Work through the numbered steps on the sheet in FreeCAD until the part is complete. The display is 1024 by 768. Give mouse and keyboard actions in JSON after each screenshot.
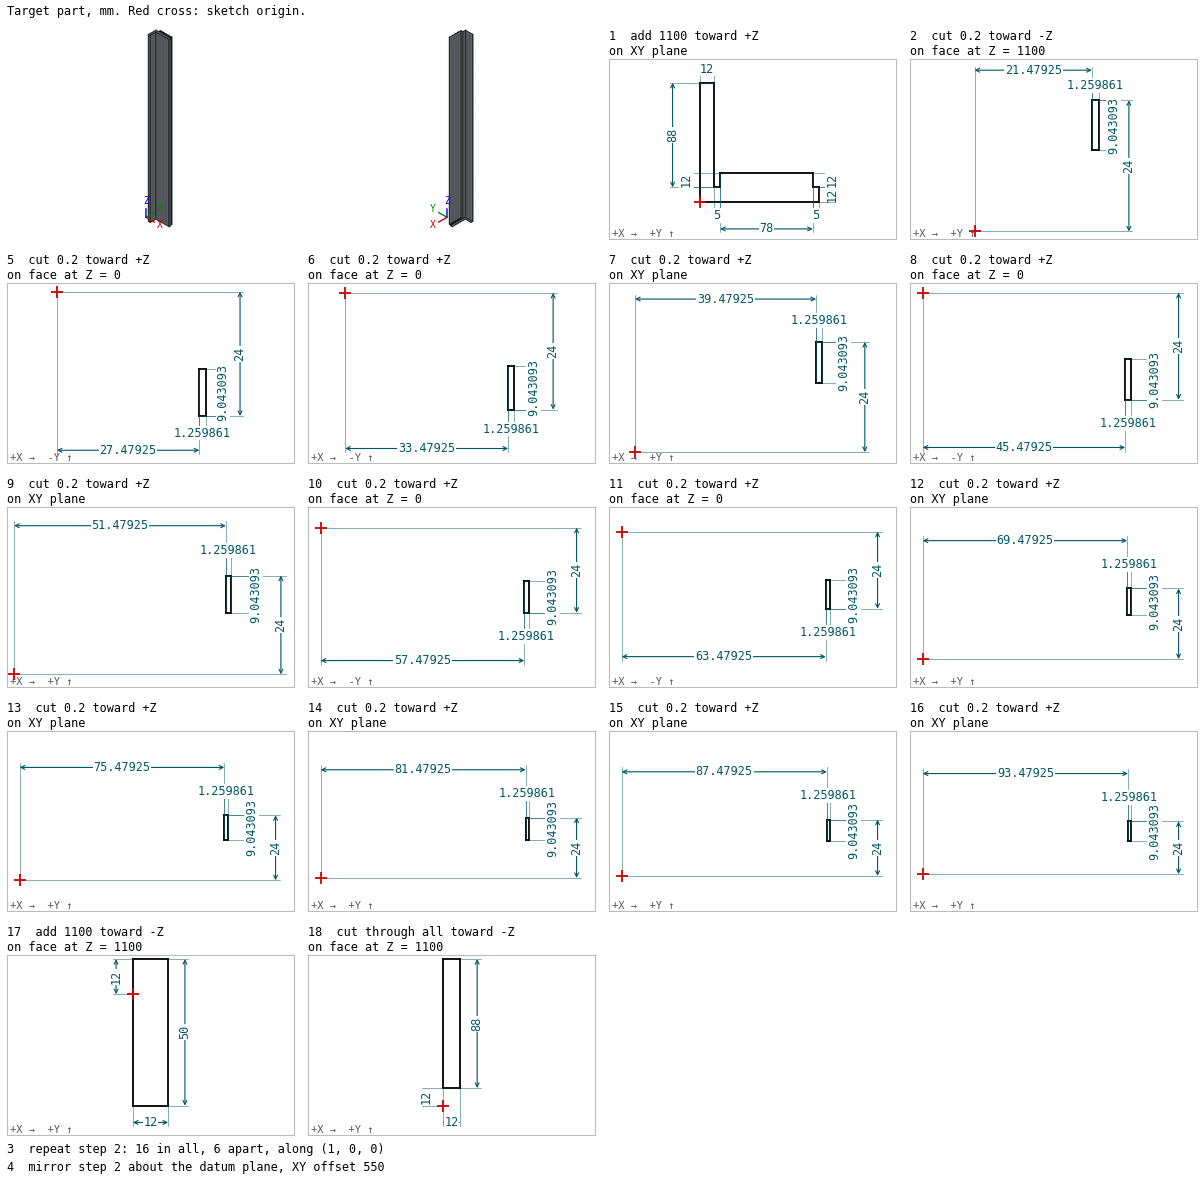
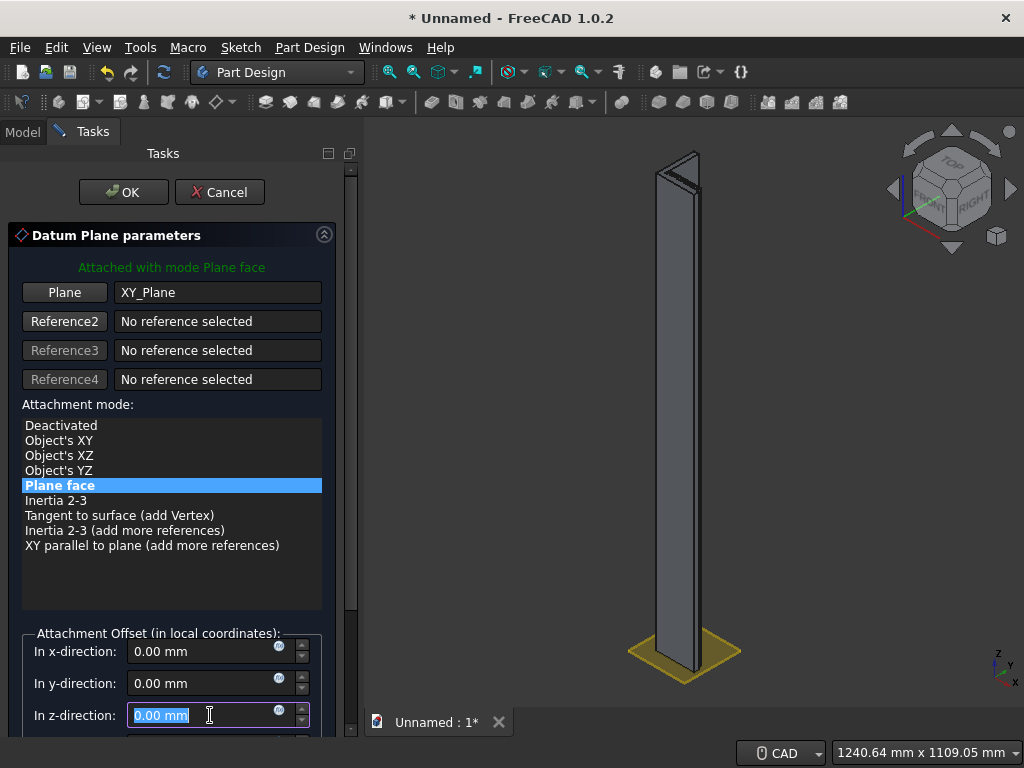
{"action": "type", "text": "550"}
{"action": "key", "text": "Tab"}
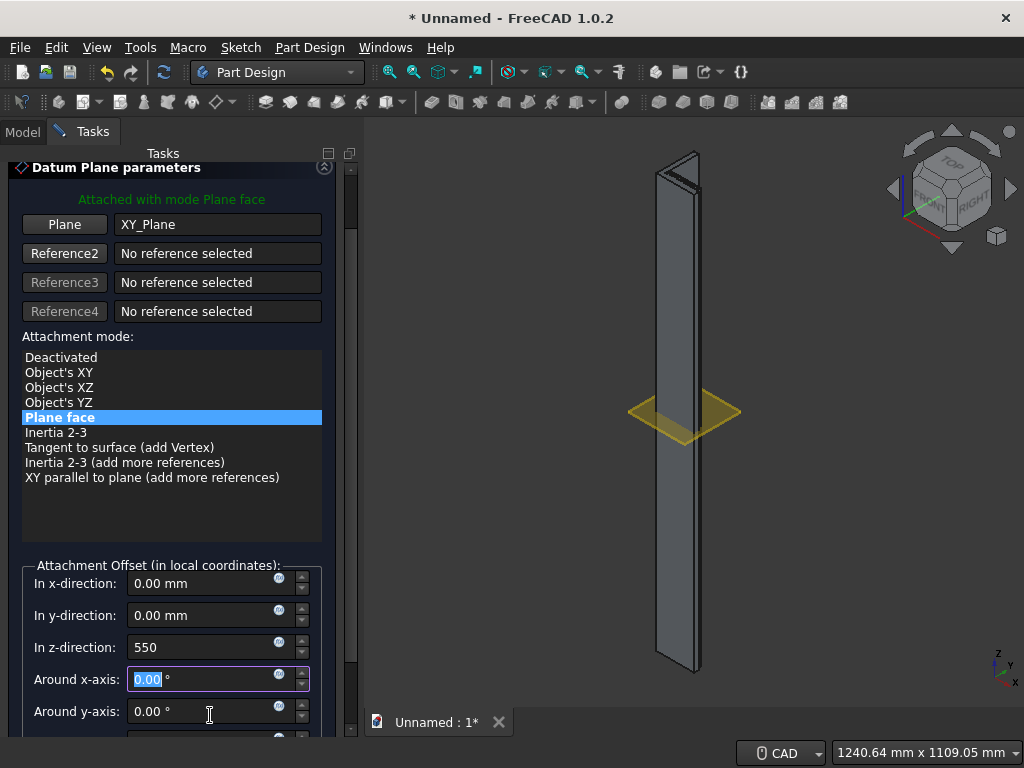
{"action": "scroll", "coordinate": [351, 450], "scroll_direction": "up", "scroll_amount": 2}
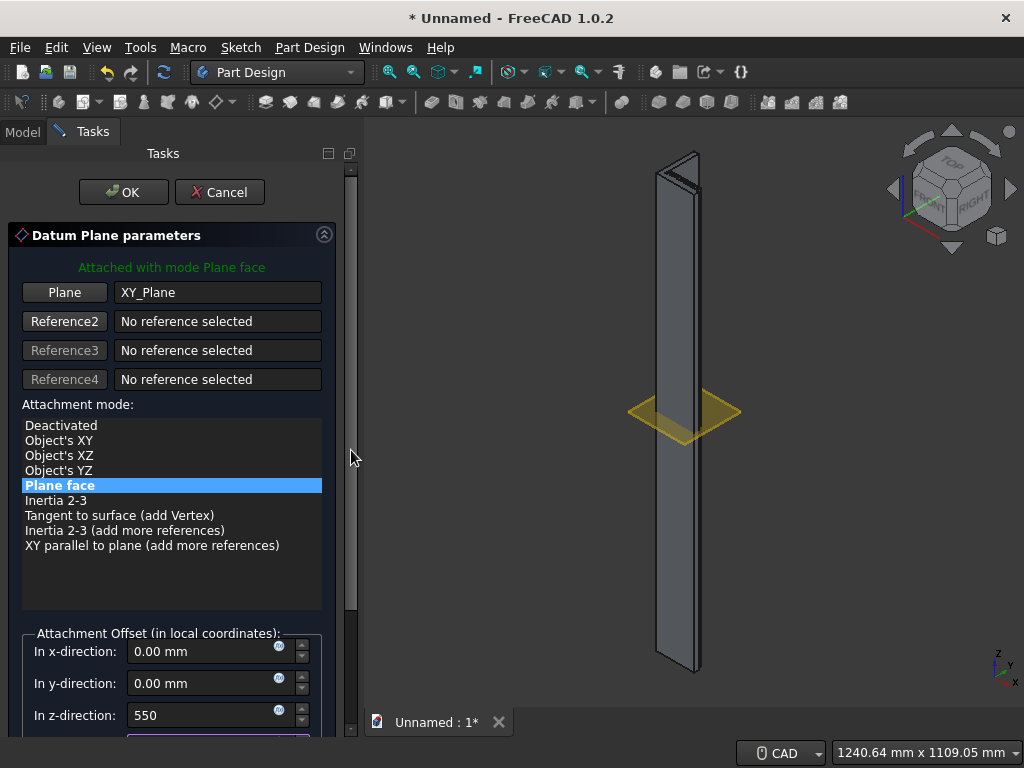
{"action": "left_click", "coordinate": [124, 192]}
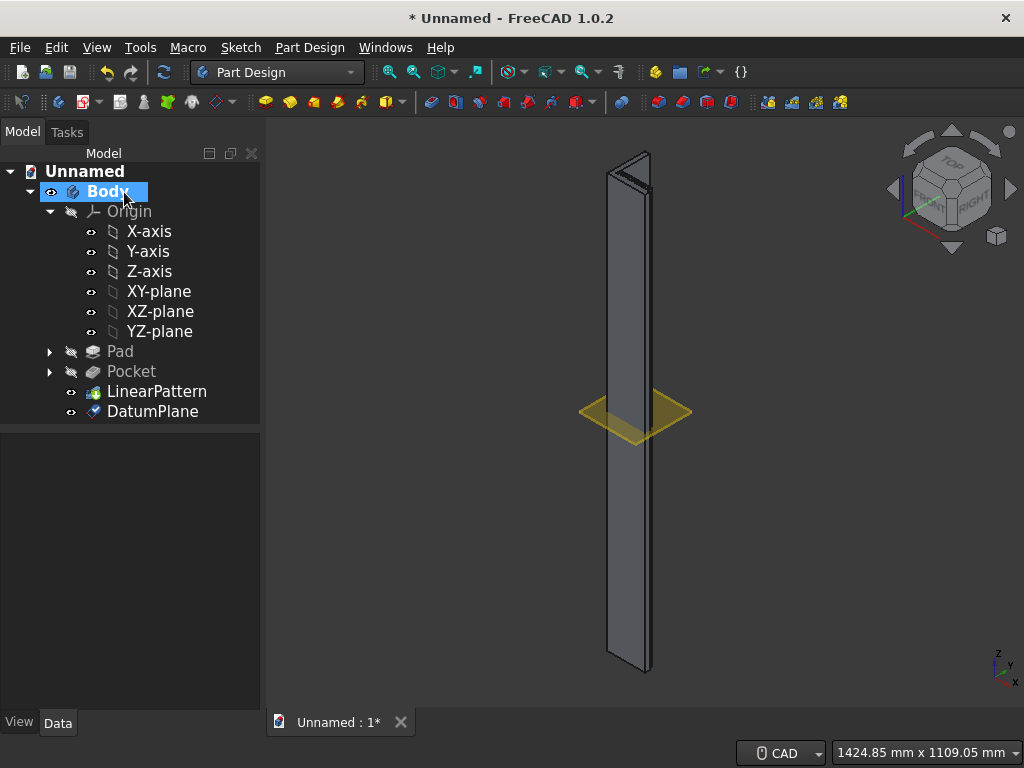
{"action": "left_click", "coordinate": [116, 372]}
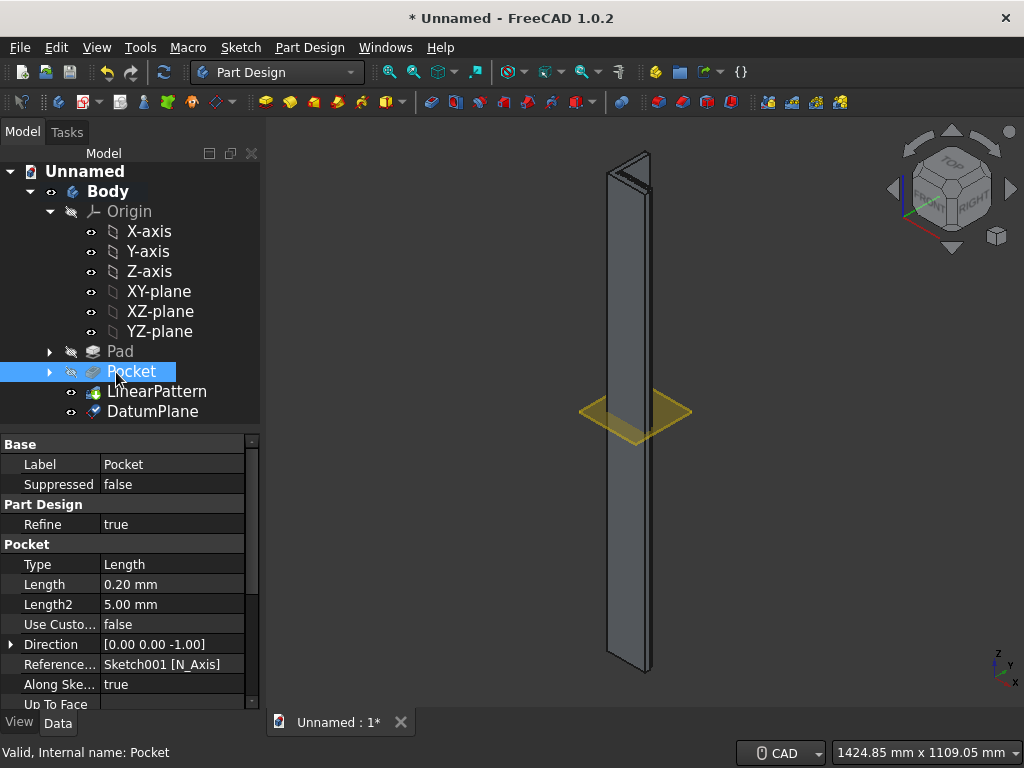
{"action": "left_click", "coordinate": [768, 102]}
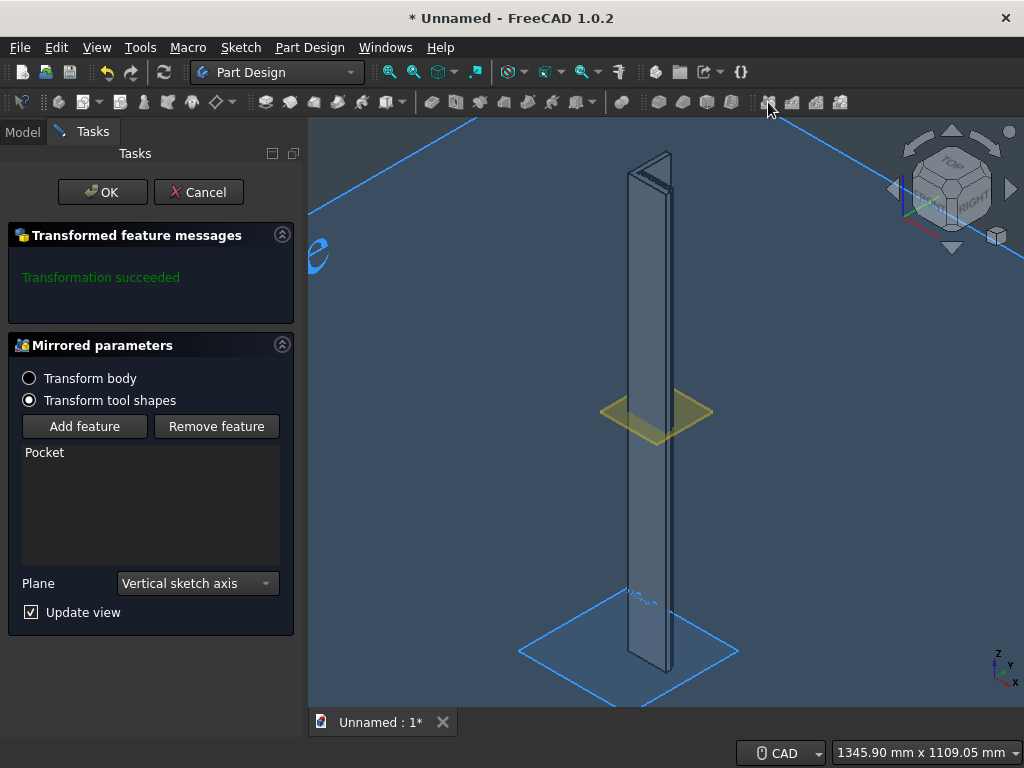
{"action": "left_click", "coordinate": [198, 584]}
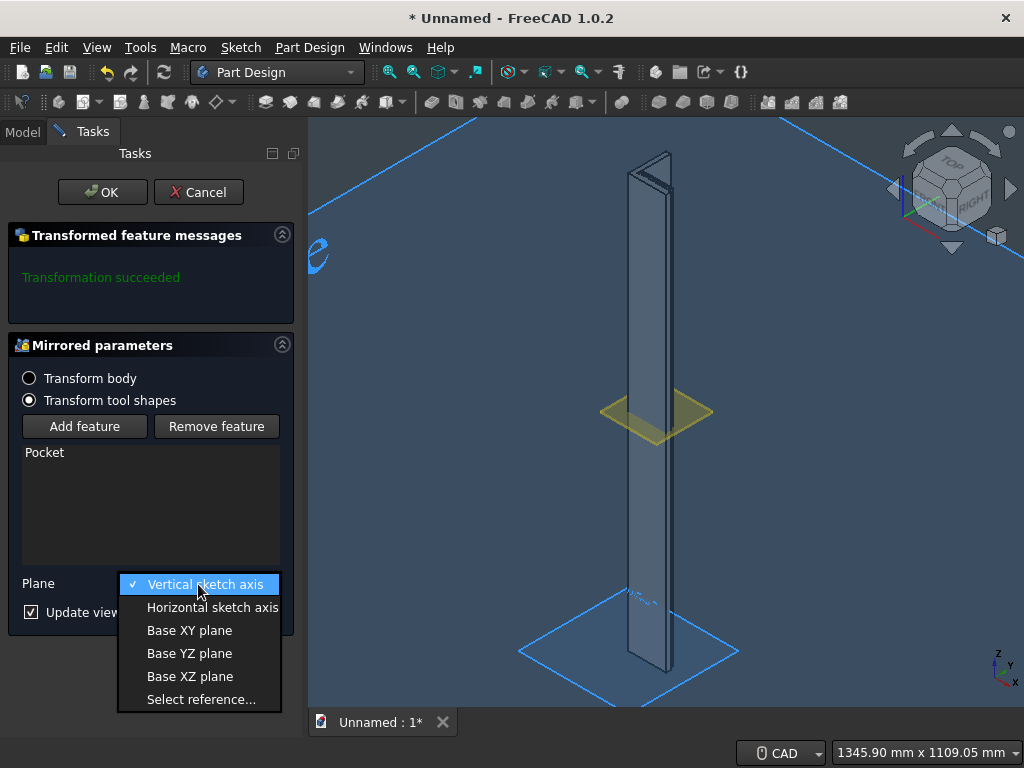
{"action": "left_click", "coordinate": [198, 700]}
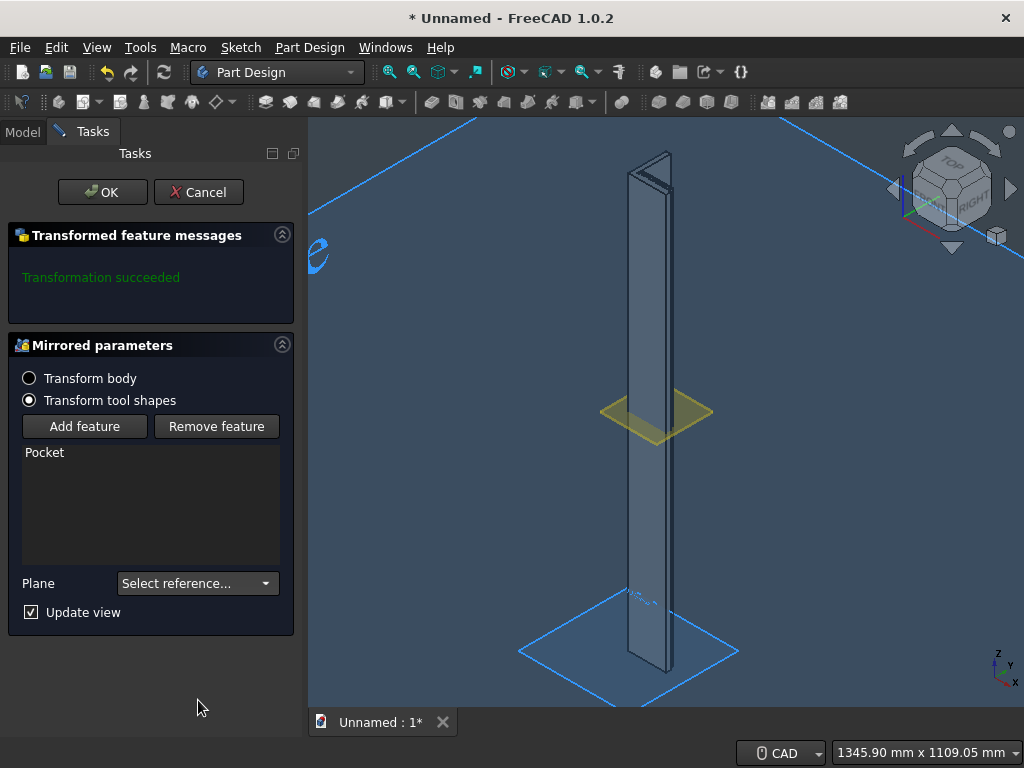
{"action": "left_click", "coordinate": [23, 131]}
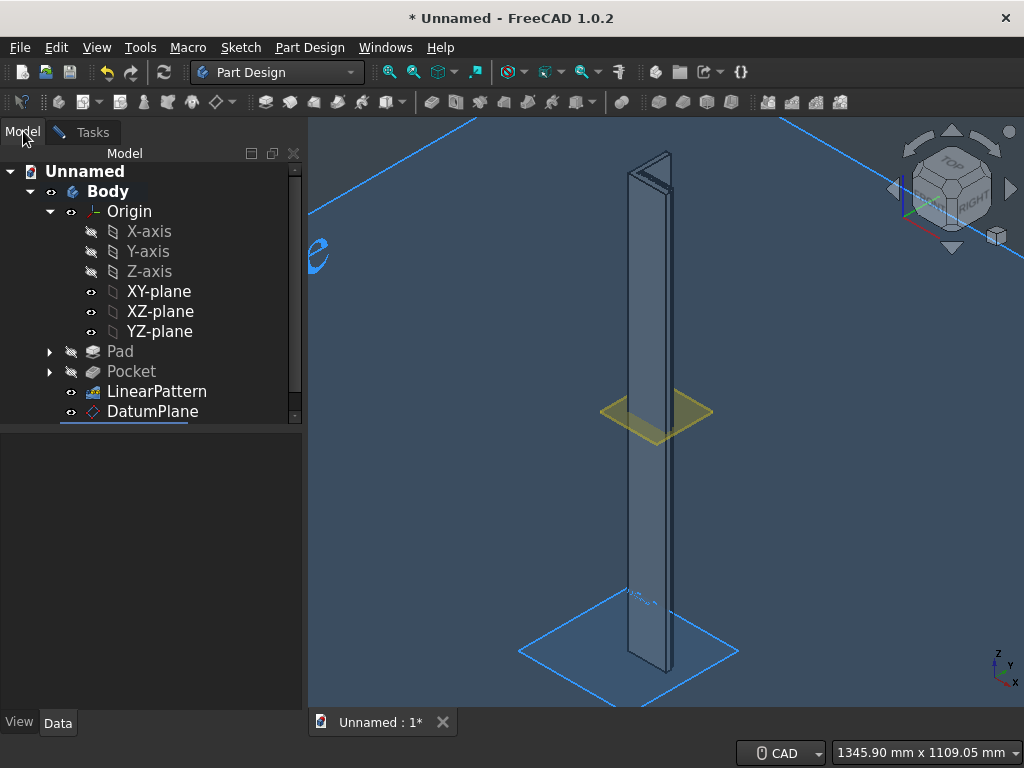
{"action": "left_click", "coordinate": [116, 412]}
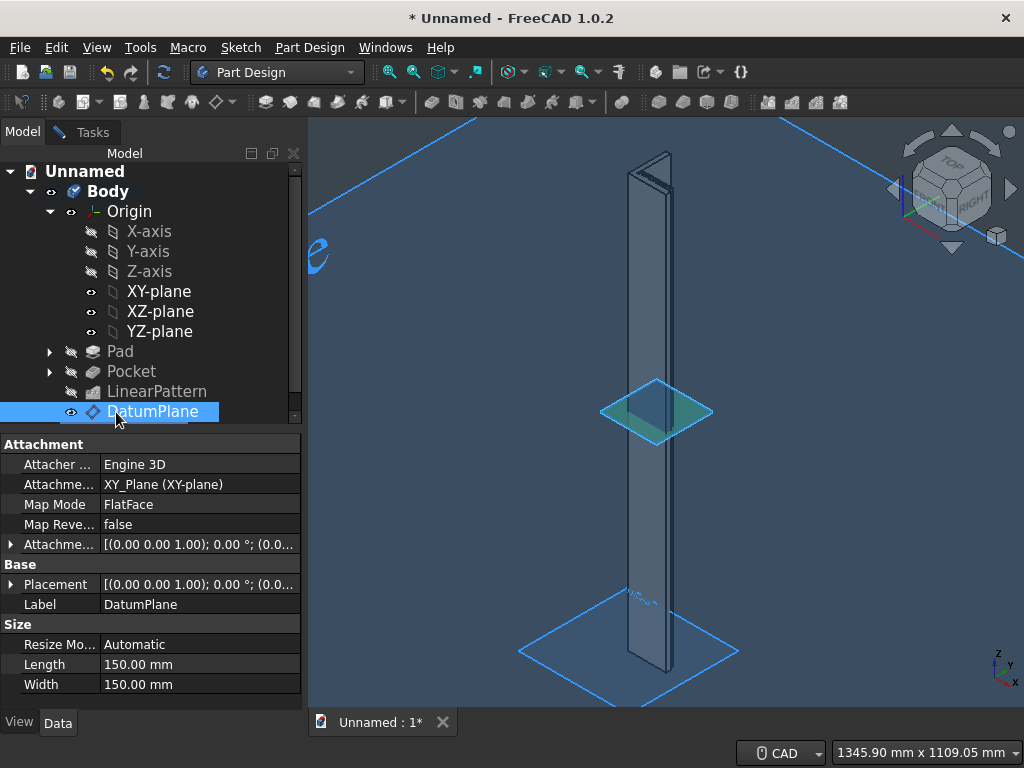
{"action": "left_click", "coordinate": [84, 131]}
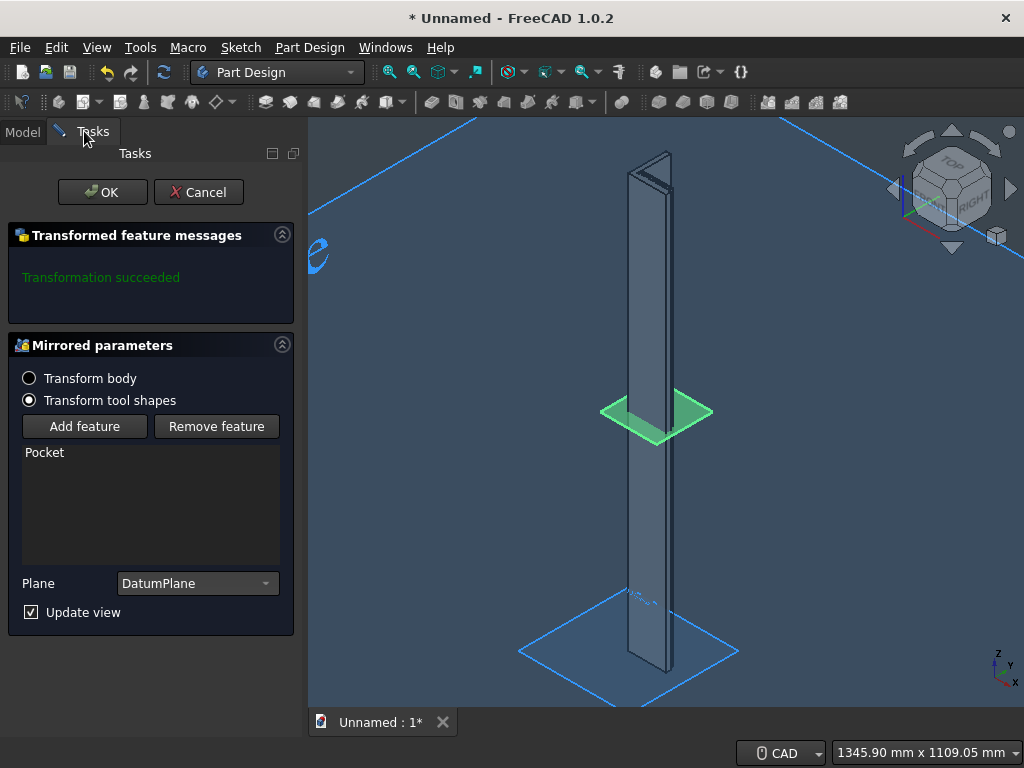
{"action": "left_click", "coordinate": [103, 192]}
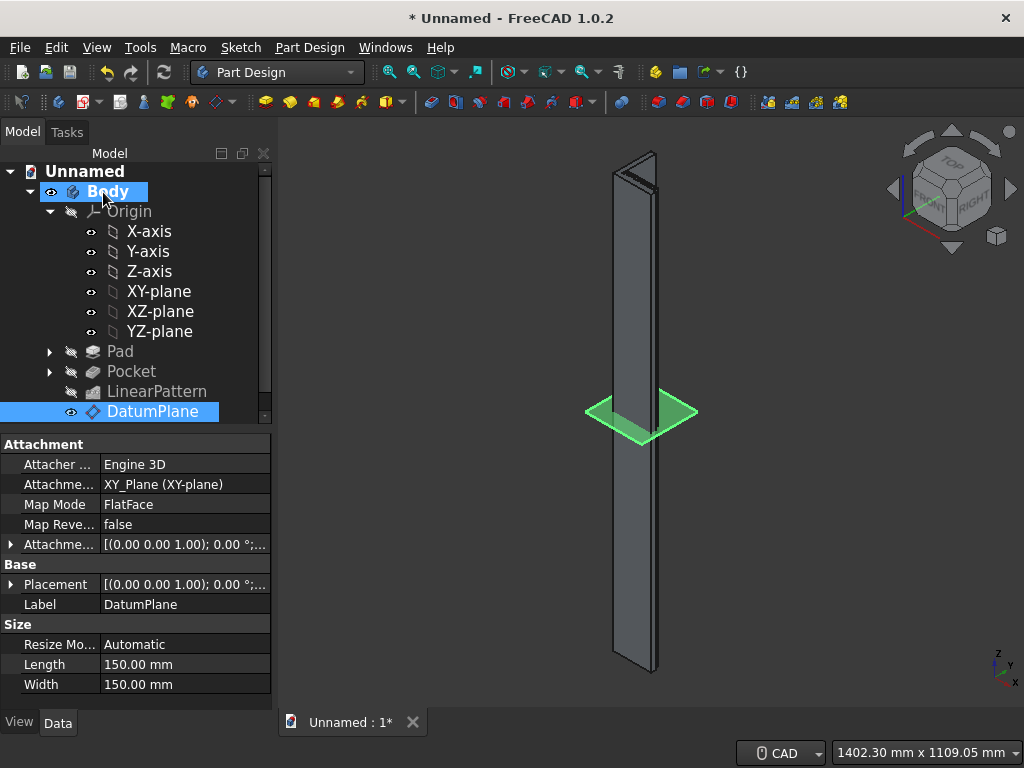
{"action": "left_click", "coordinate": [116, 412]}
{"action": "key", "text": "space"}